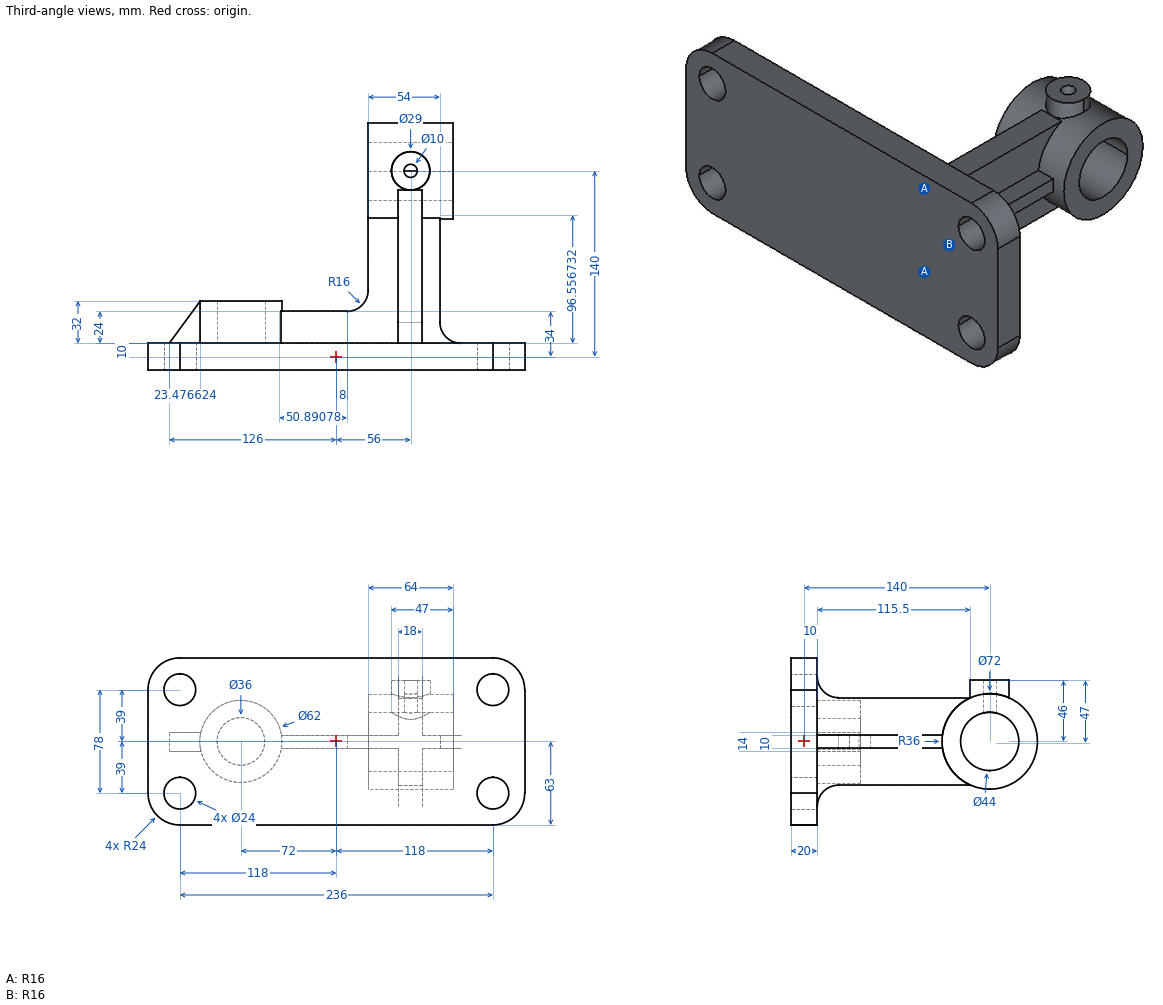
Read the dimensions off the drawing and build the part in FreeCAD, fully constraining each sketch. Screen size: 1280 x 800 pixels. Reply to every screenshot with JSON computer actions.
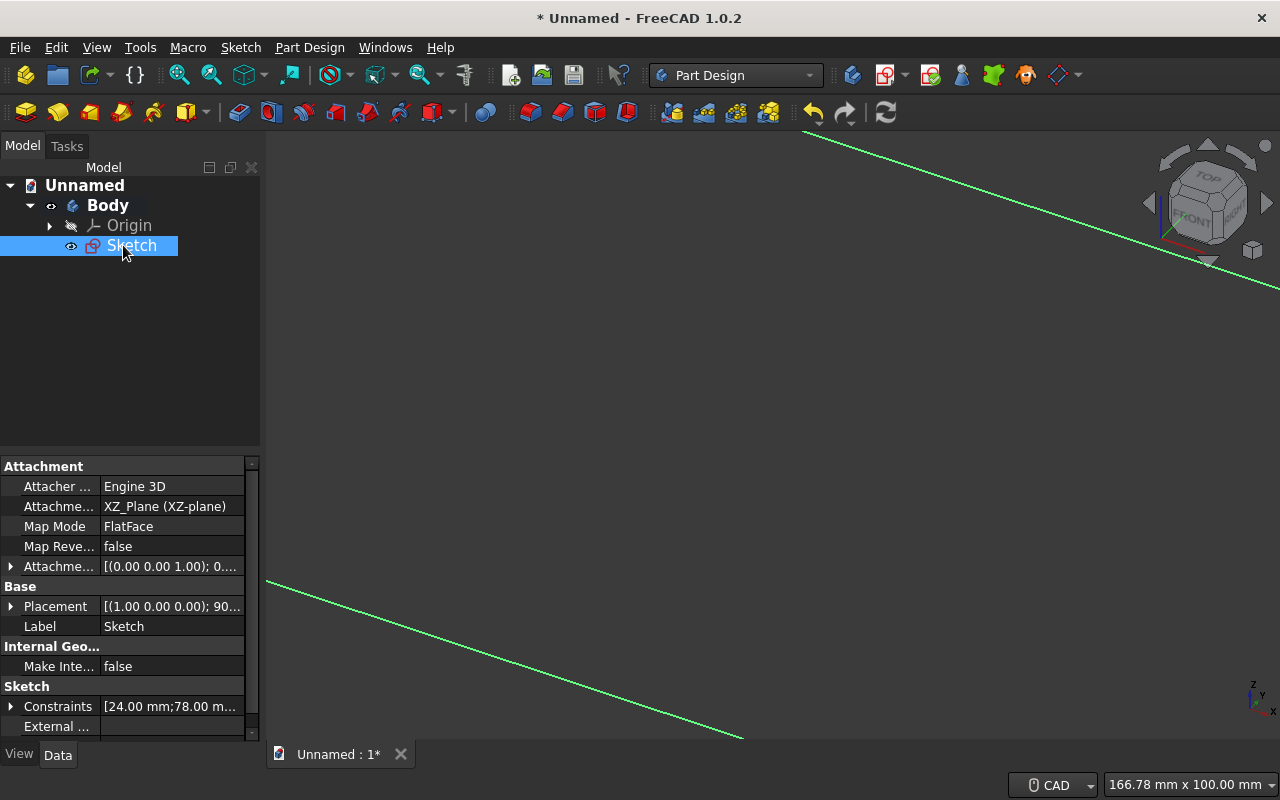
{"action": "left_click", "coordinate": [26, 112]}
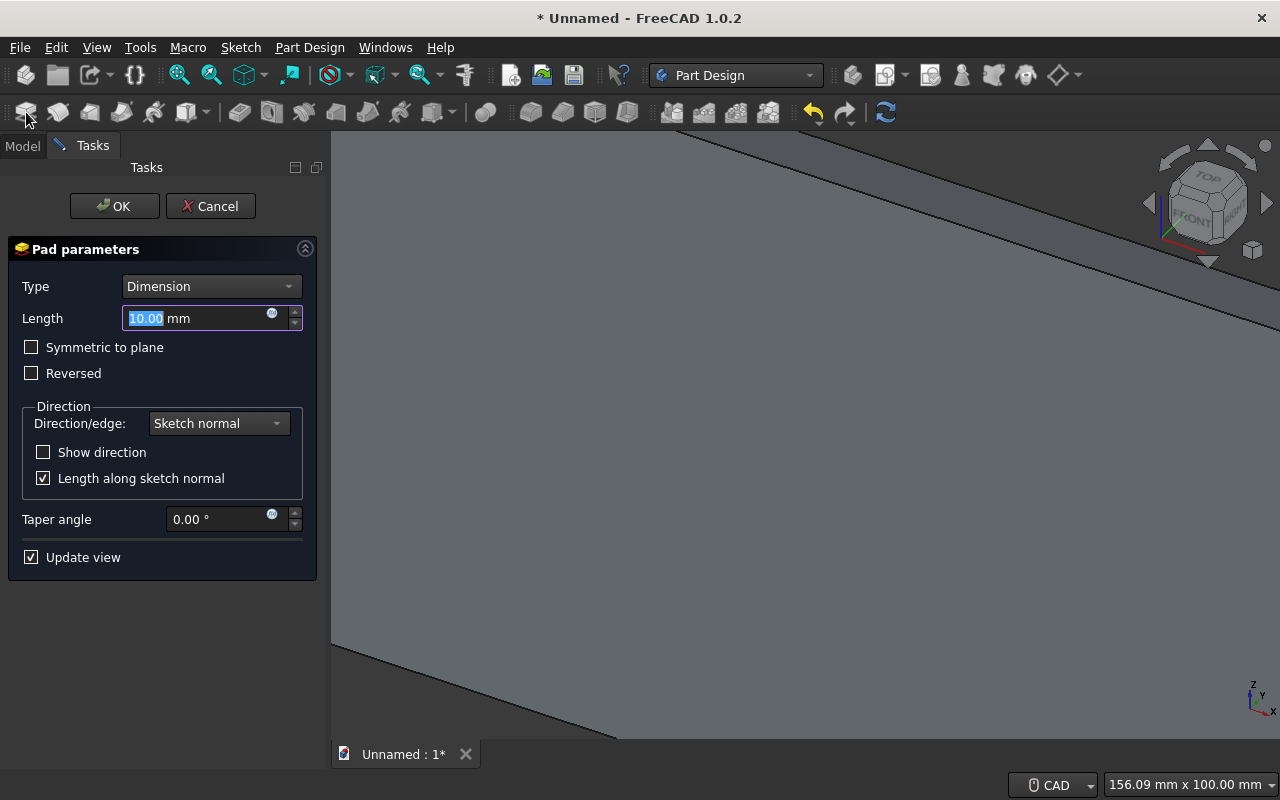
{"action": "type", "text": "20"}
{"action": "key", "text": "Tab"}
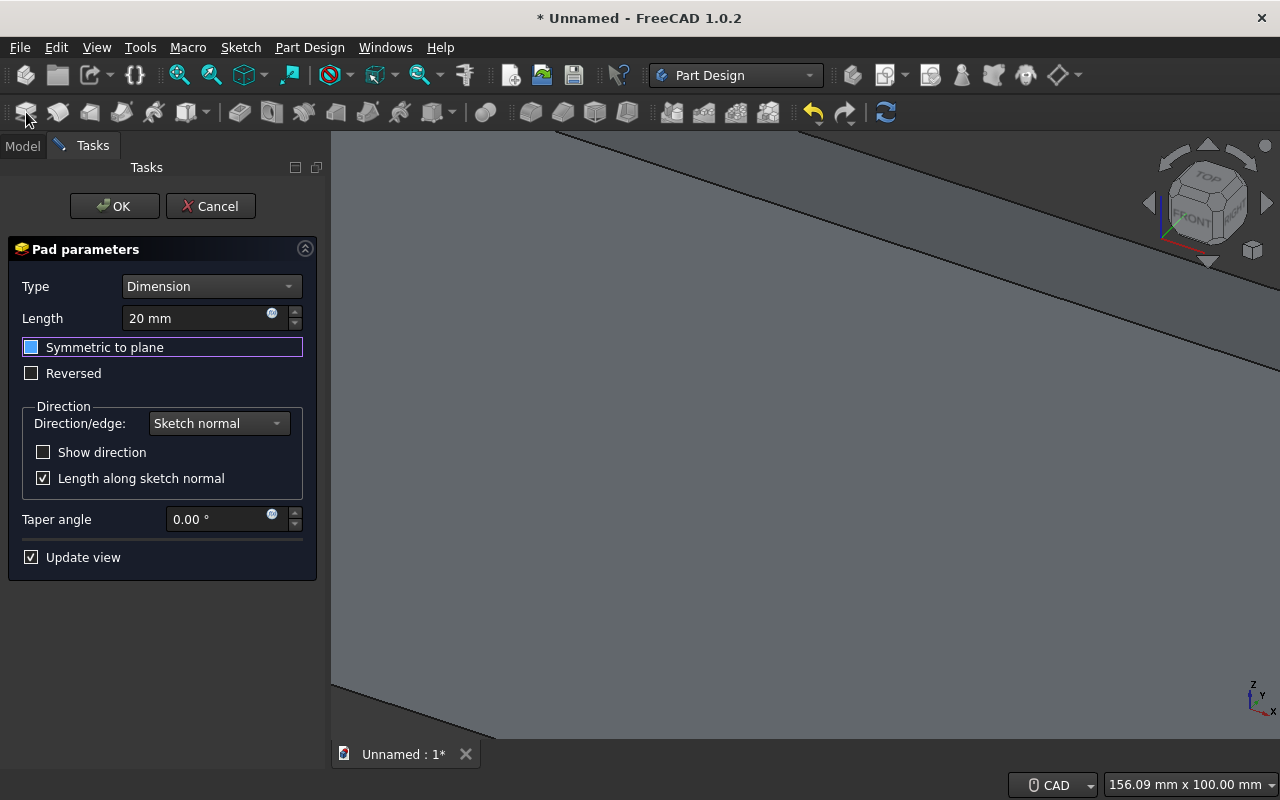
{"action": "left_click", "coordinate": [30, 347]}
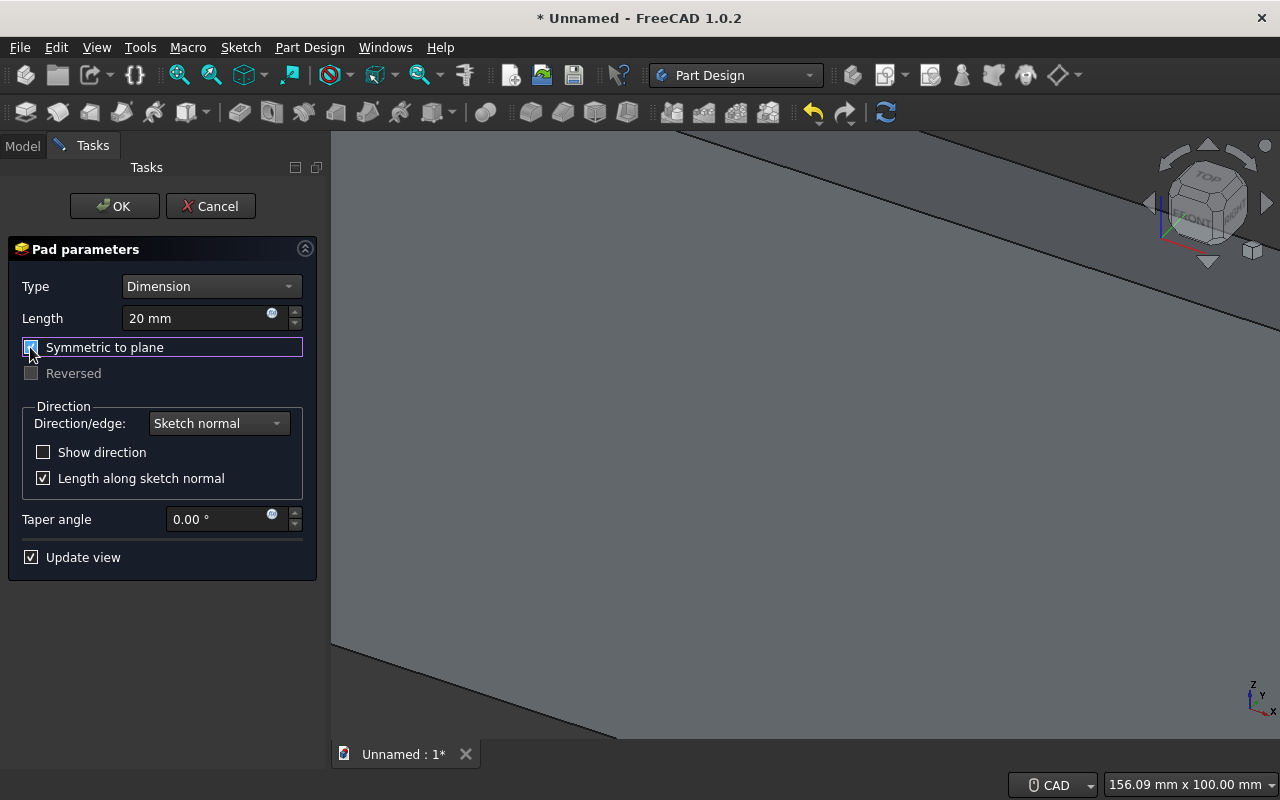
{"action": "left_click", "coordinate": [115, 206]}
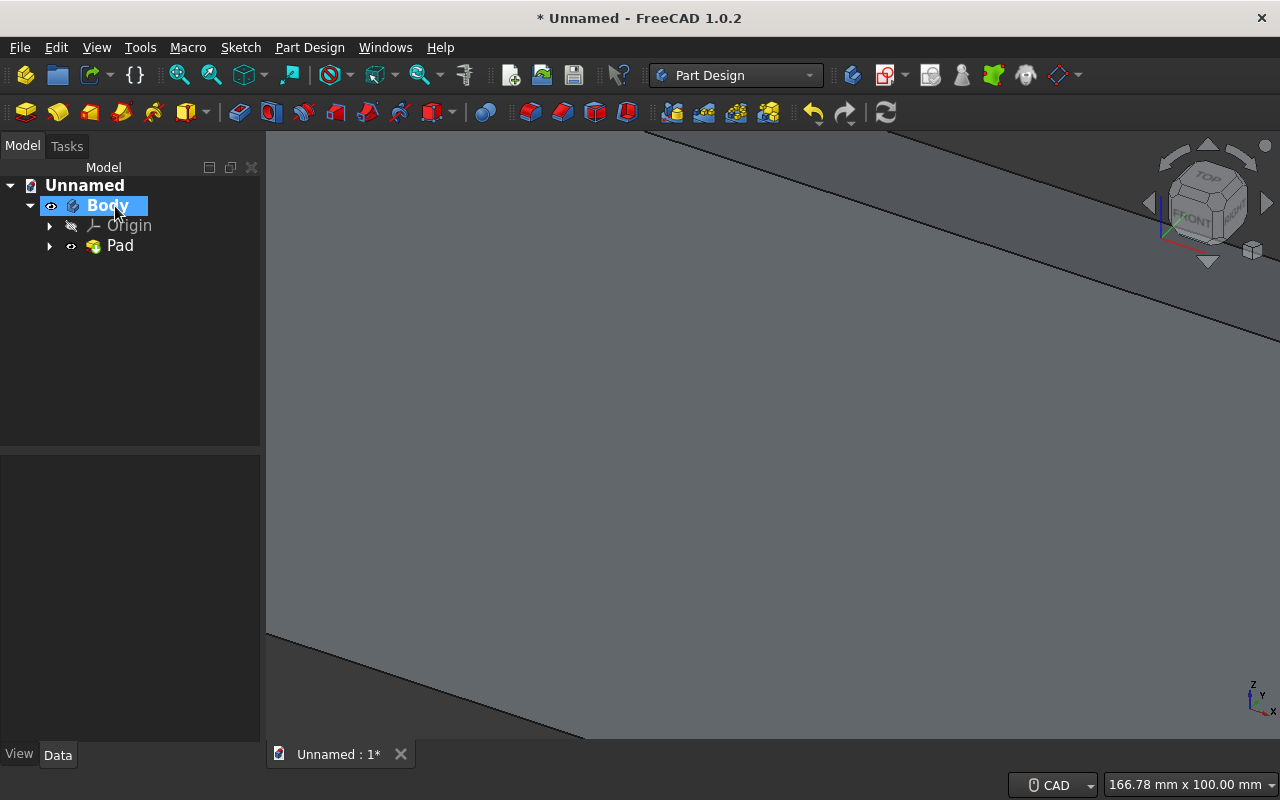
{"action": "left_click", "coordinate": [180, 76]}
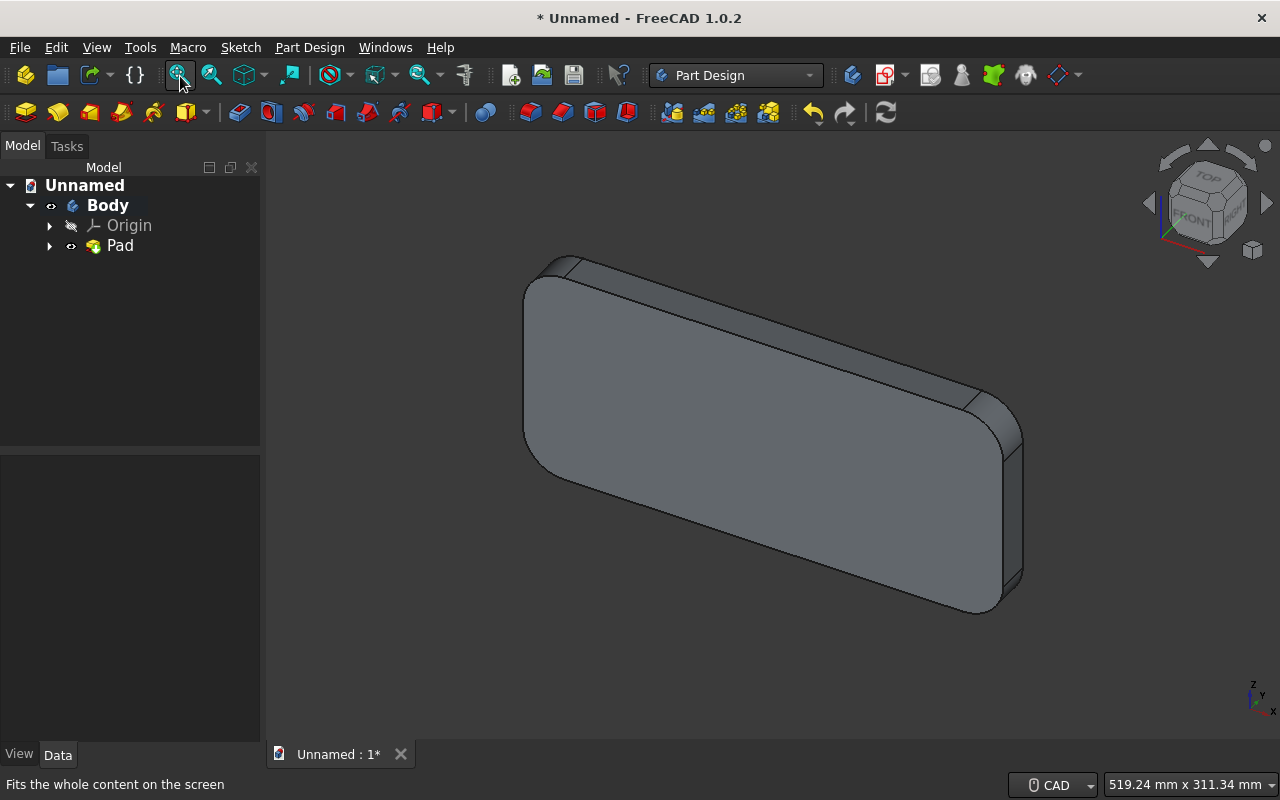
{"action": "key", "text": "4"}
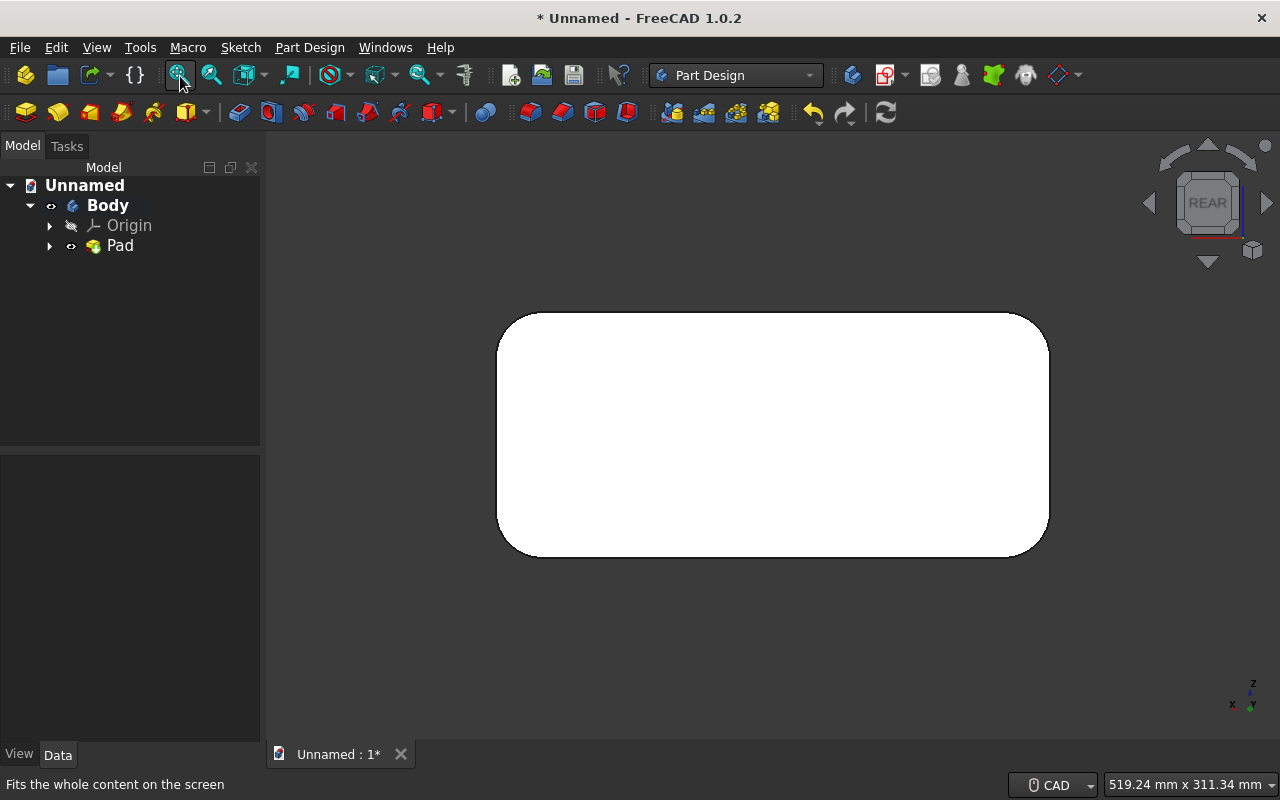
{"action": "left_click", "coordinate": [694, 434]}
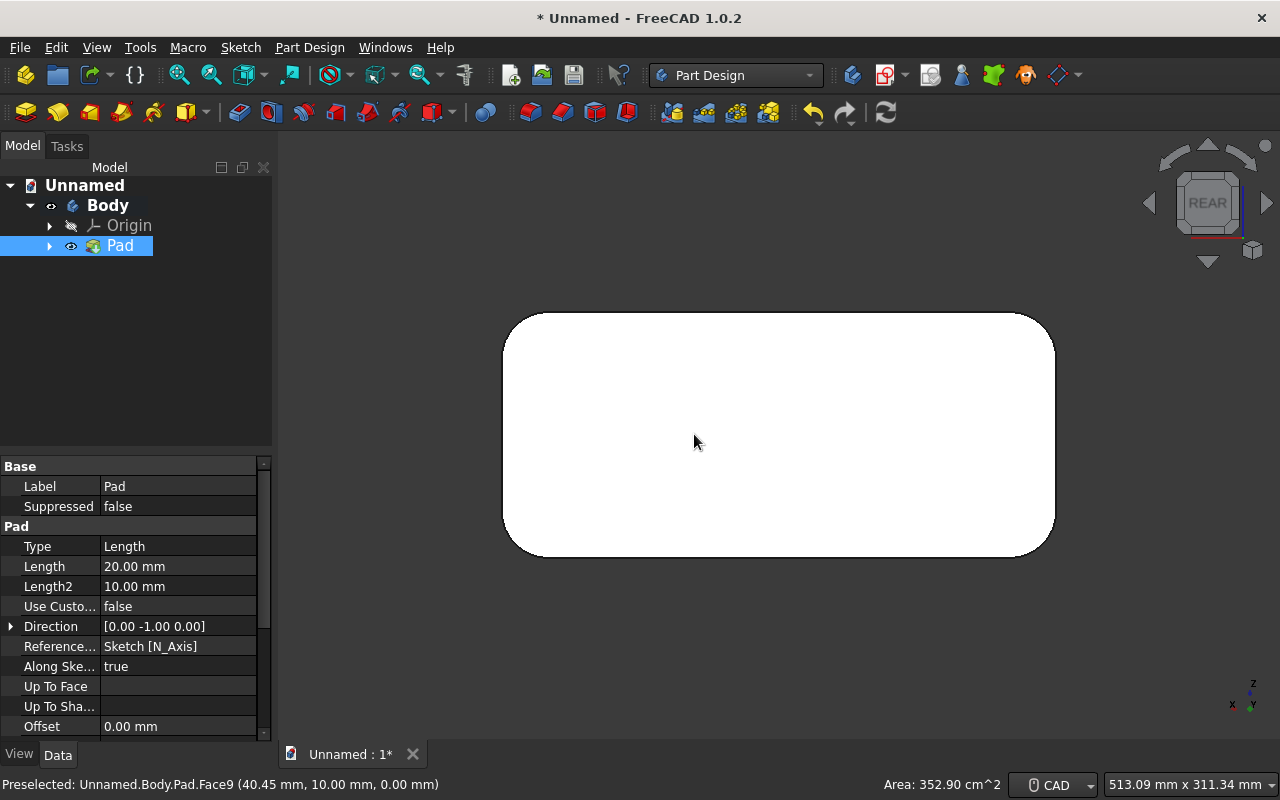
{"action": "left_click", "coordinate": [886, 76]}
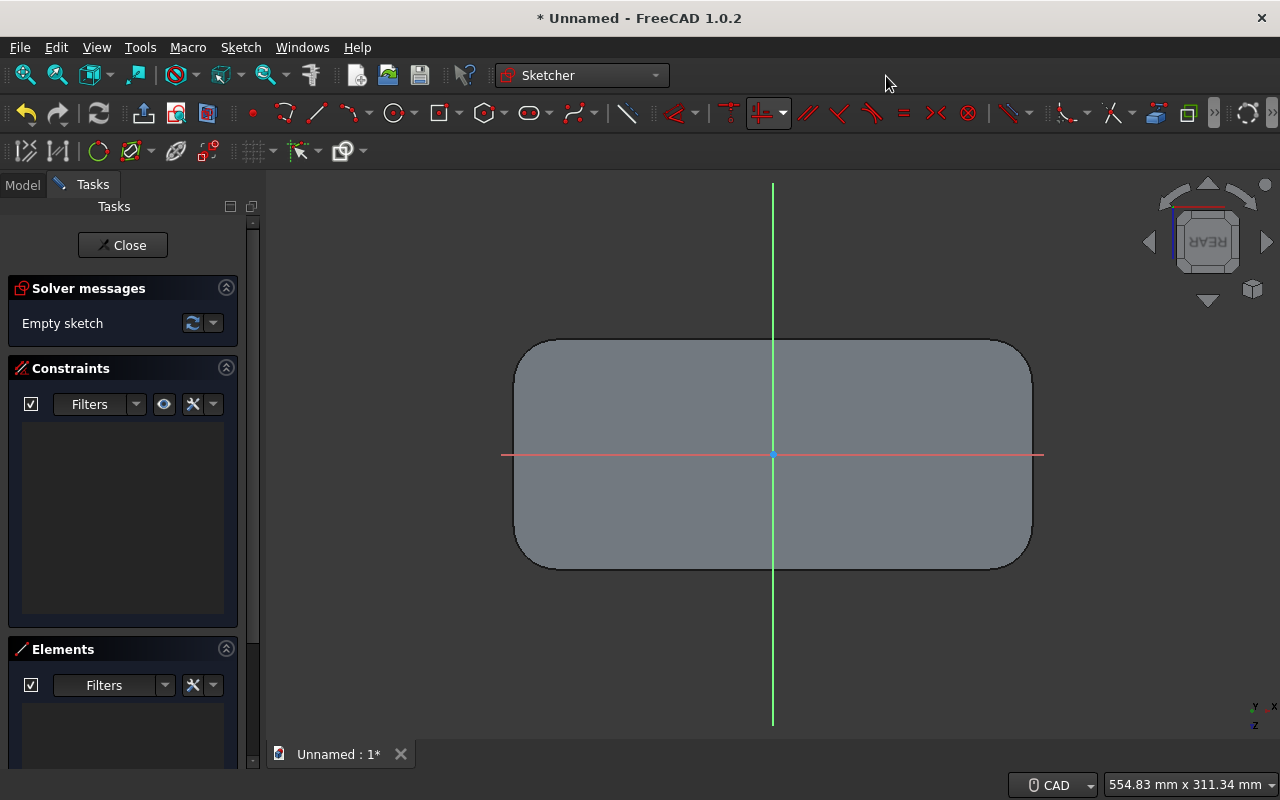
{"action": "scroll", "coordinate": [668, 455], "scroll_direction": "up", "scroll_amount": 6}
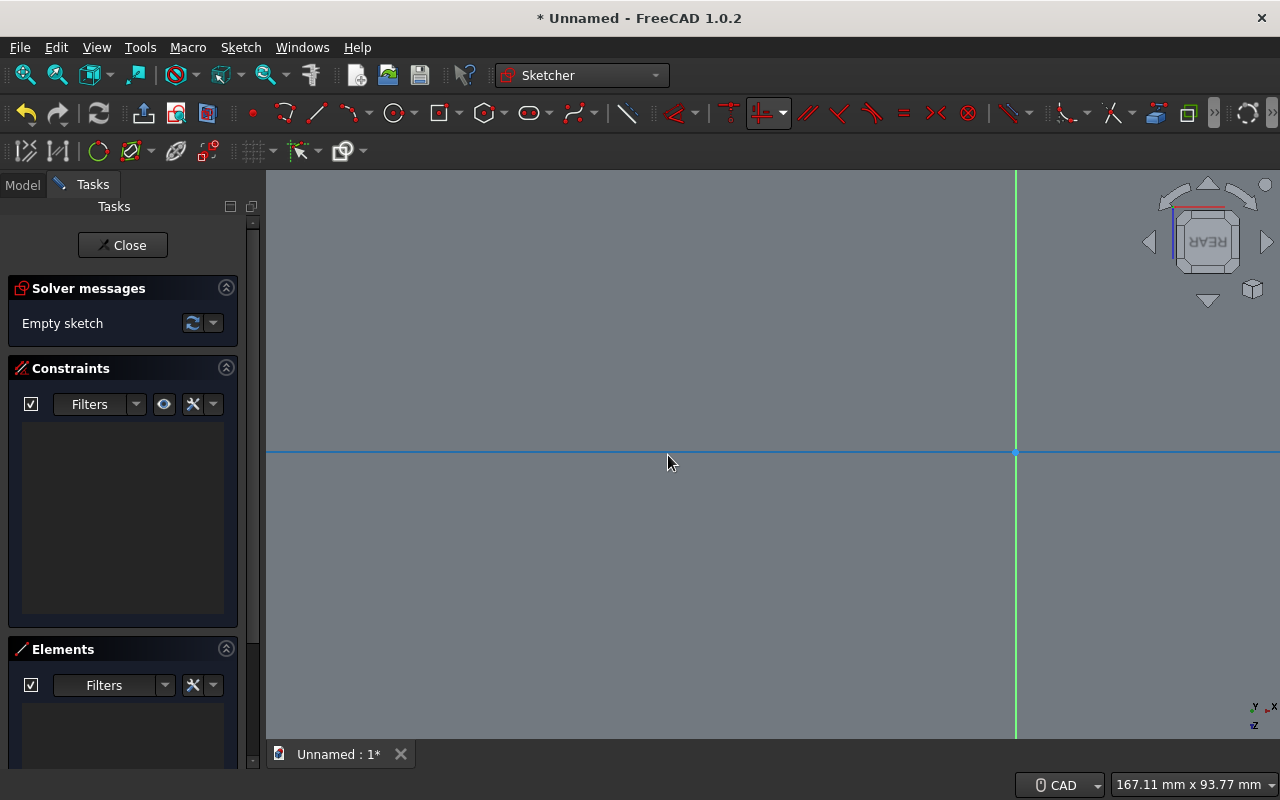
{"action": "left_click", "coordinate": [394, 114]}